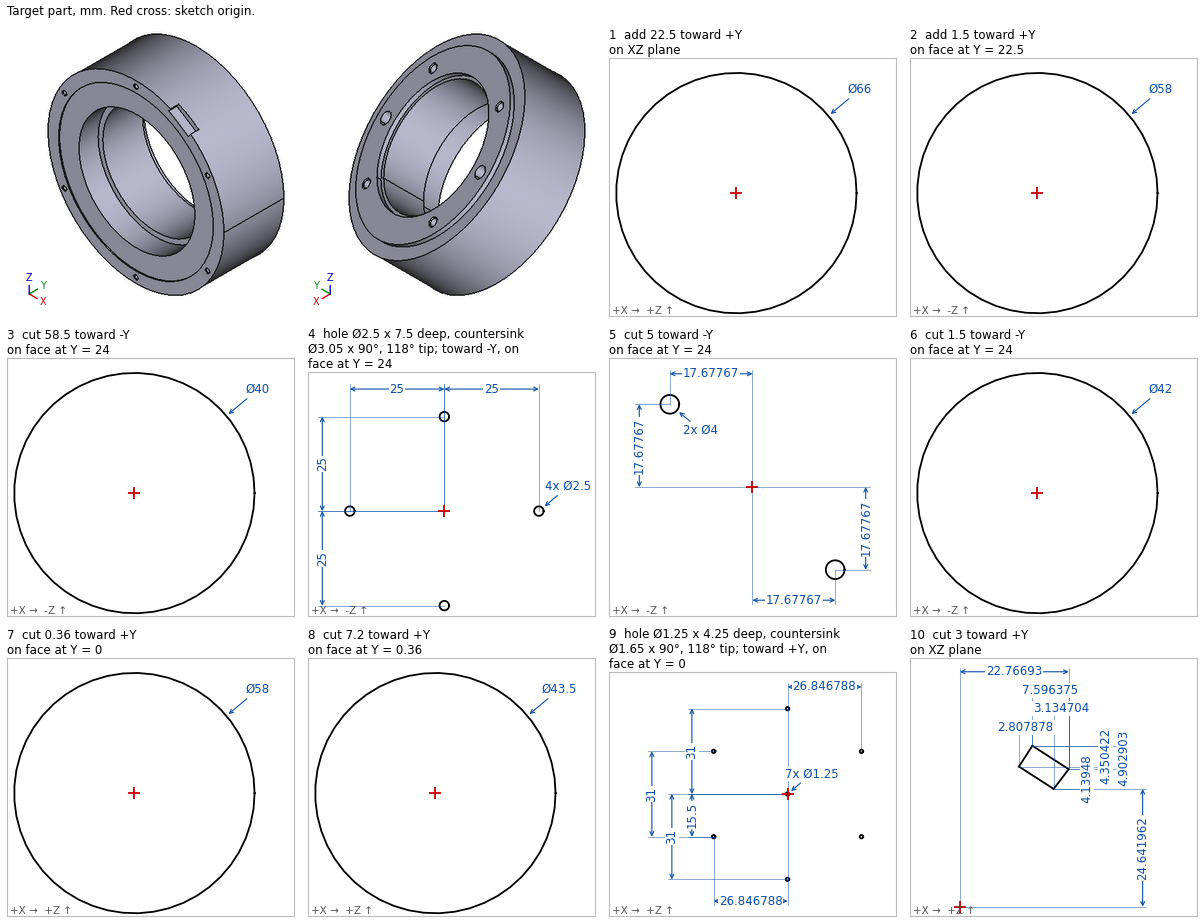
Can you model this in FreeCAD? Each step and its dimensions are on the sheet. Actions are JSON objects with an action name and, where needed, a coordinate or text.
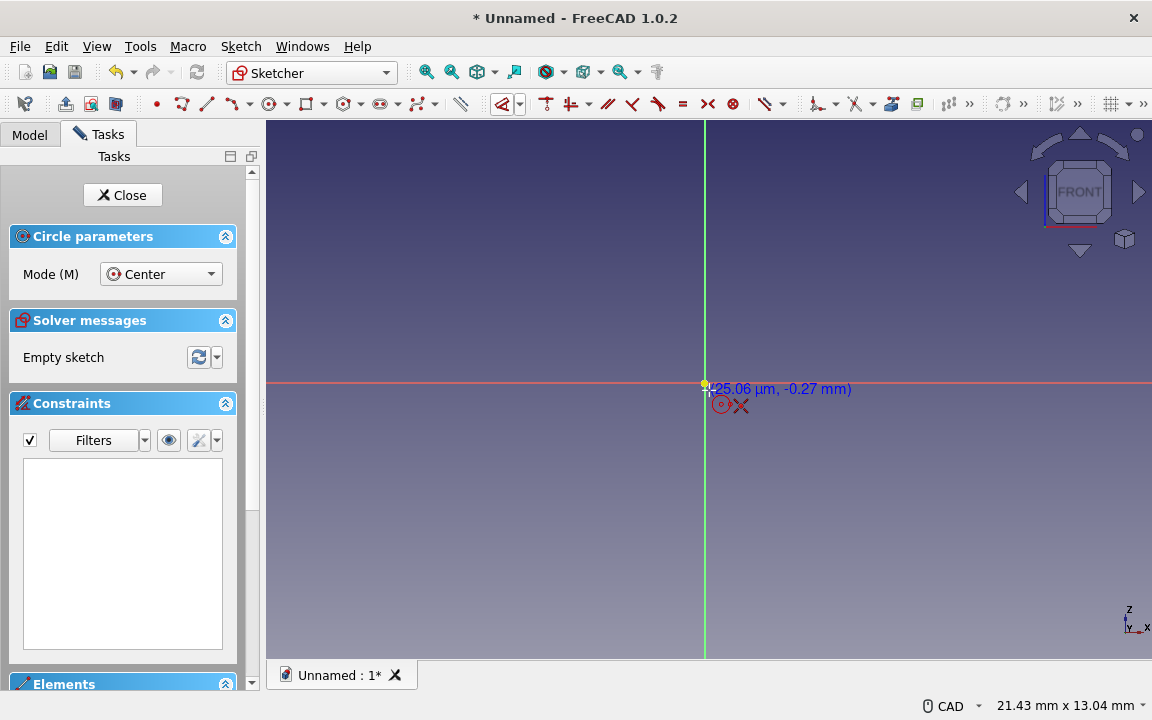
{"action": "scroll", "coordinate": [630, 391], "scroll_direction": "down", "scroll_amount": 10}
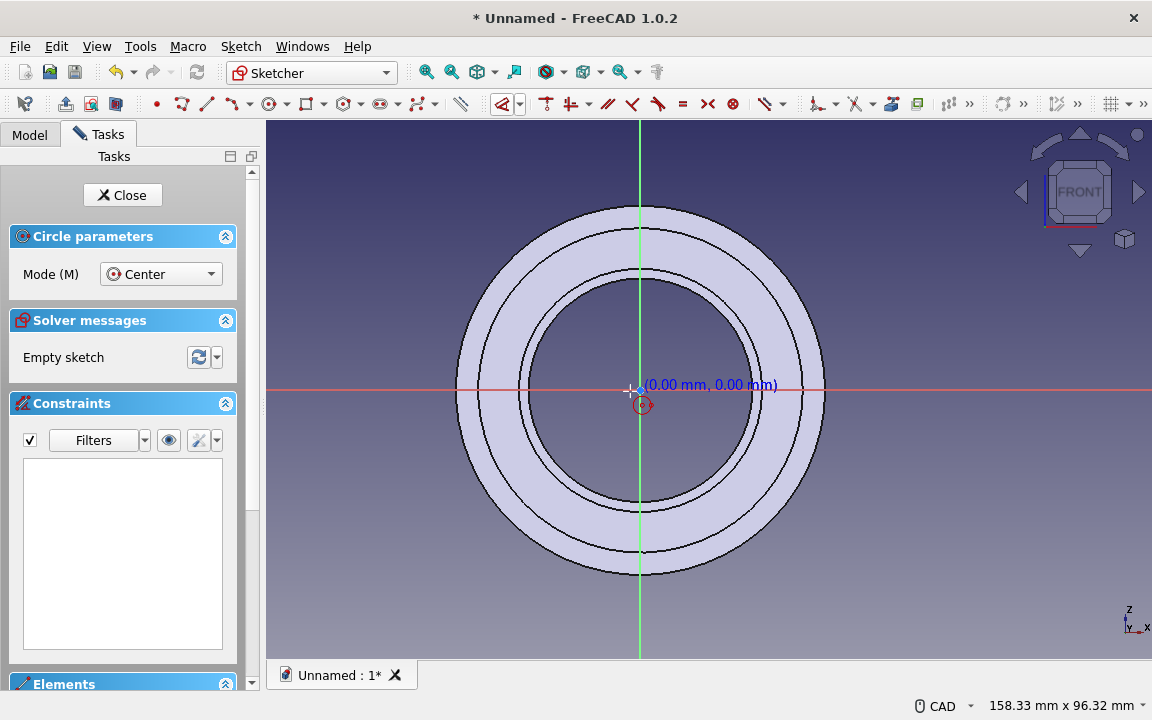
{"action": "left_click", "coordinate": [640, 390]}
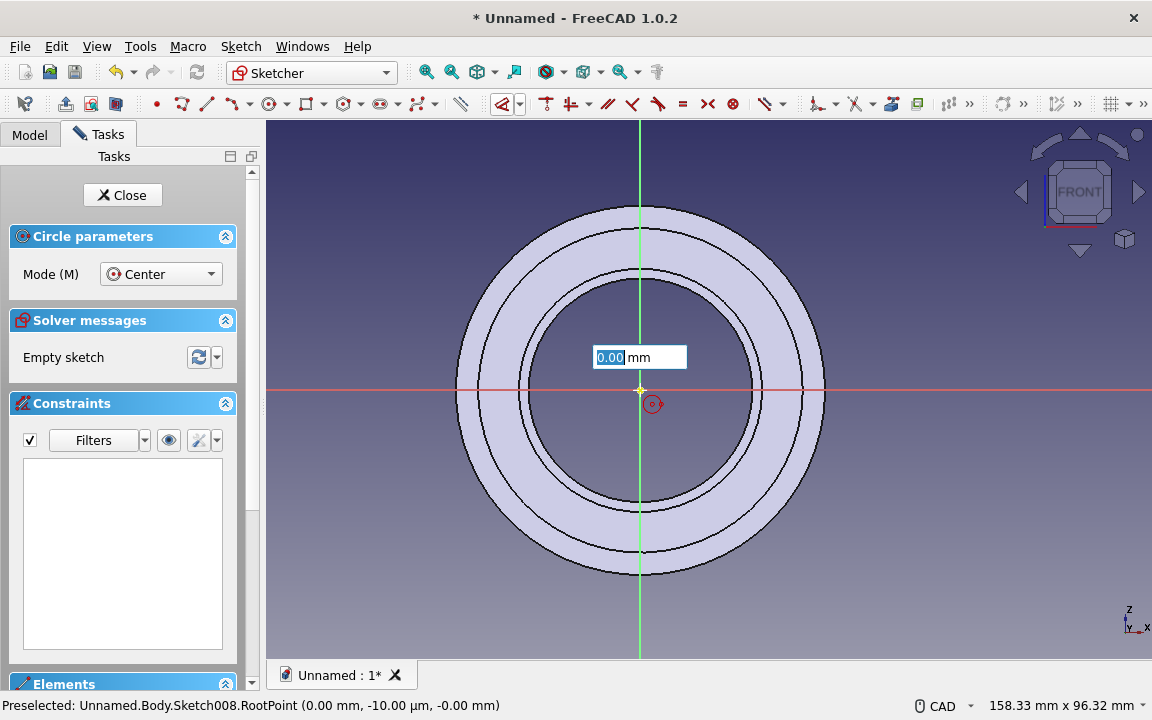
{"action": "scroll", "coordinate": [643, 388], "scroll_direction": "up", "scroll_amount": 10}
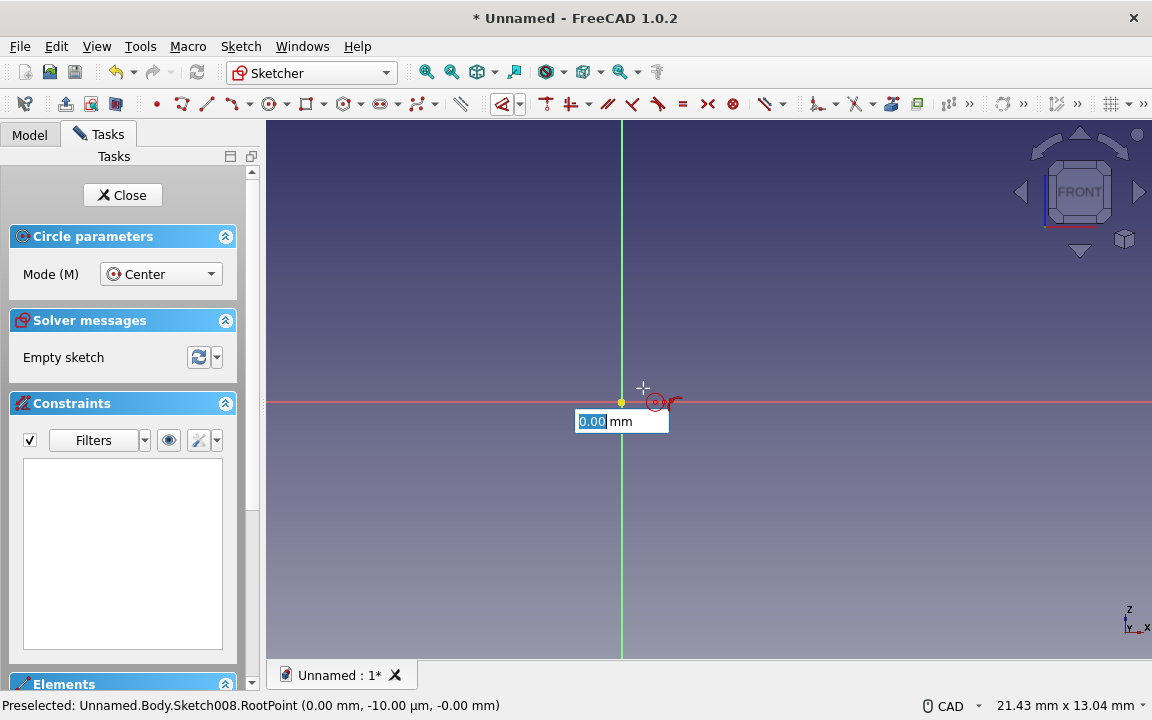
{"action": "left_click", "coordinate": [640, 384]}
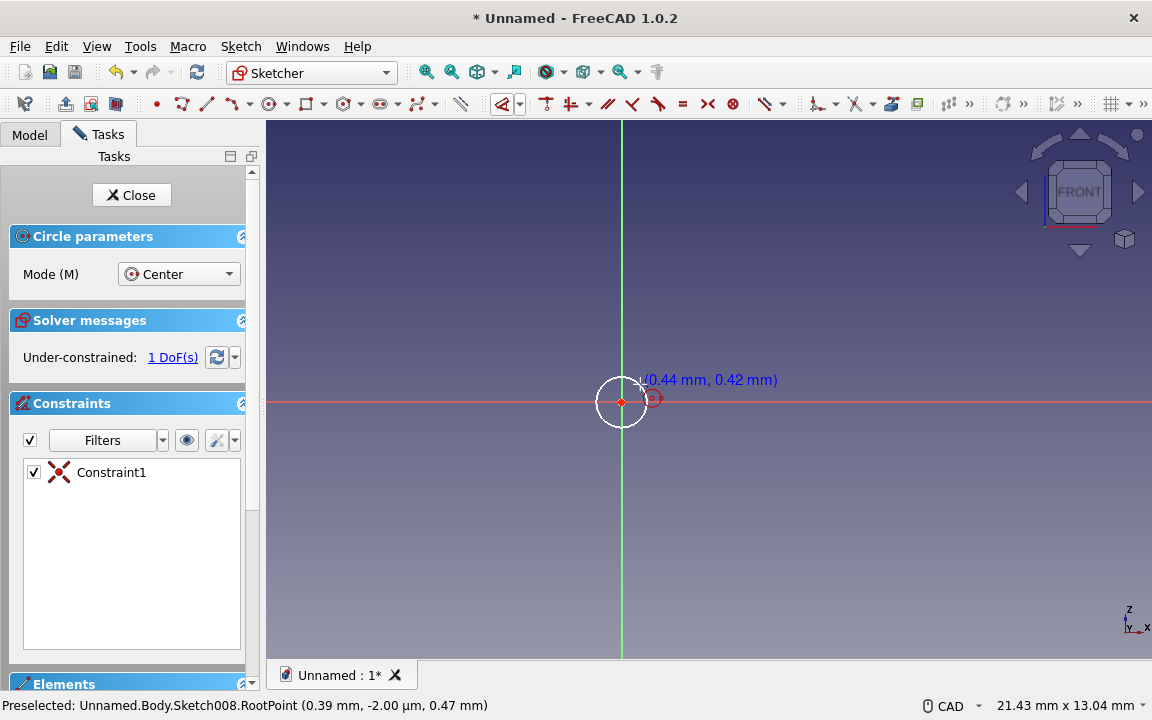
{"action": "scroll", "coordinate": [643, 387], "scroll_direction": "down", "scroll_amount": 10}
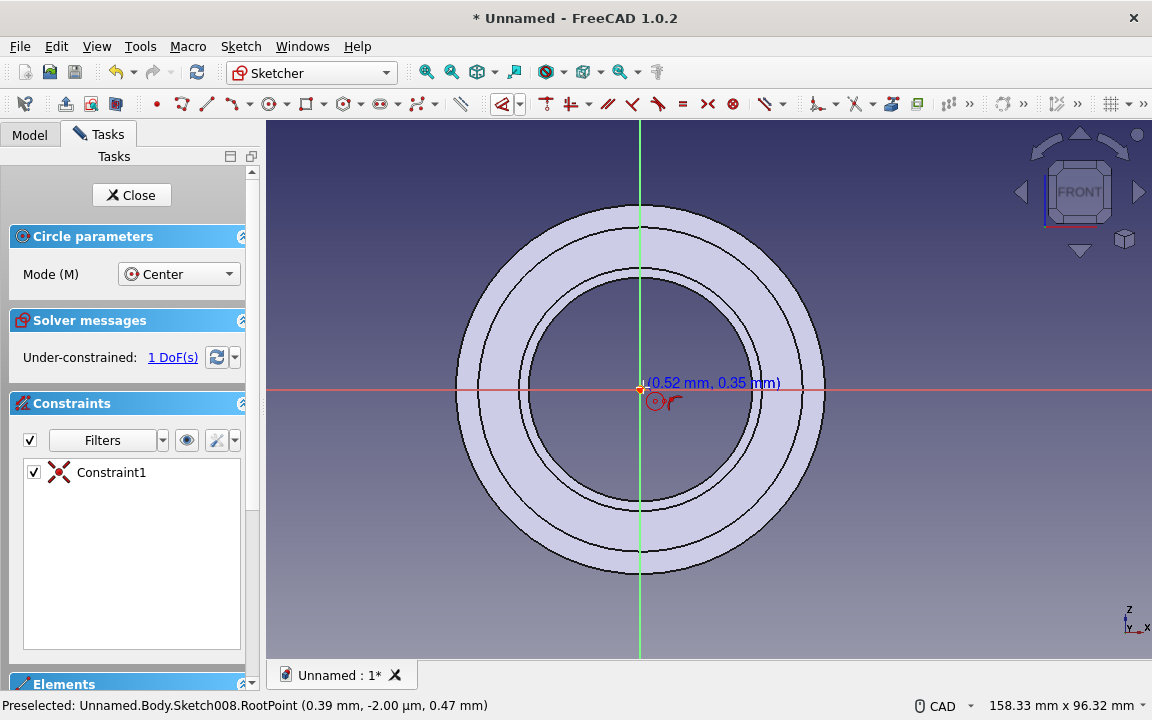
{"action": "scroll", "coordinate": [640, 563], "scroll_direction": "up", "scroll_amount": 10}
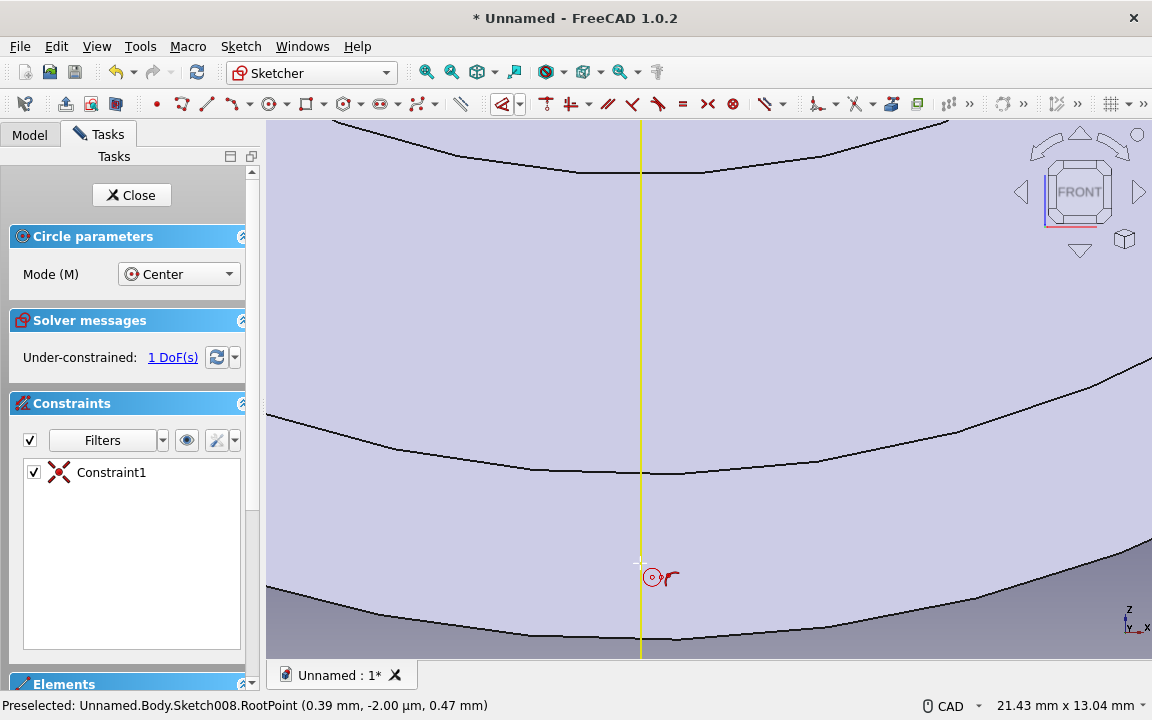
{"action": "scroll", "coordinate": [640, 564], "scroll_direction": "down", "scroll_amount": 10}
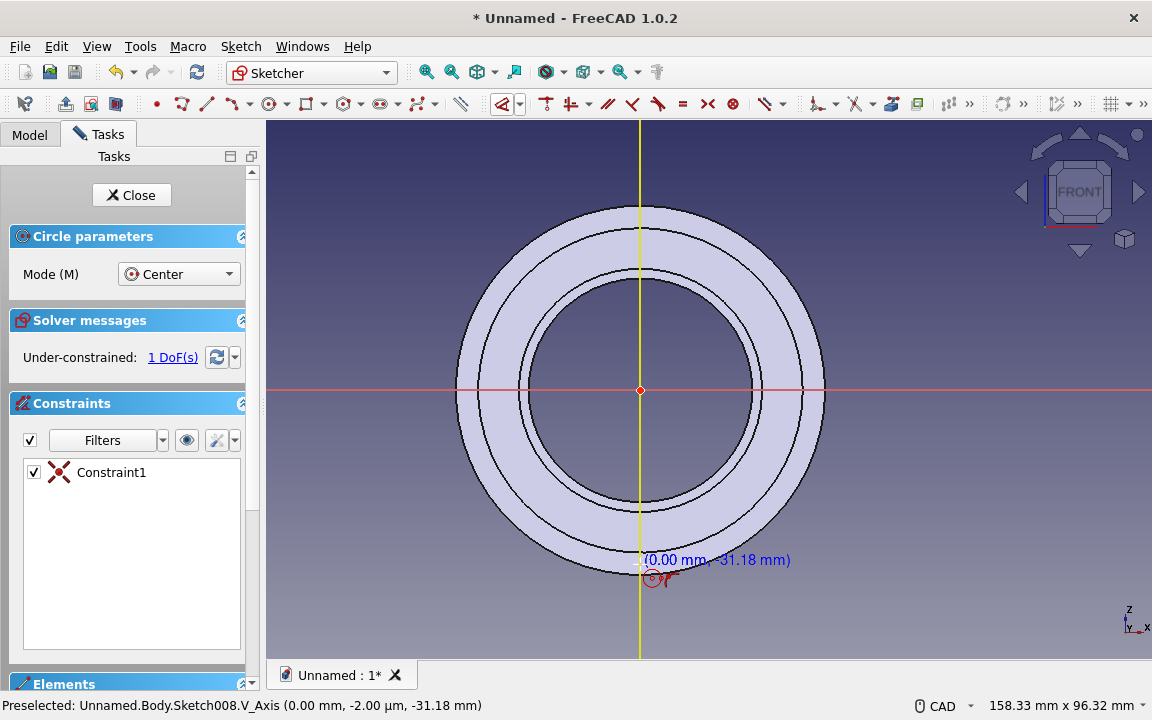
{"action": "left_click", "coordinate": [640, 564]}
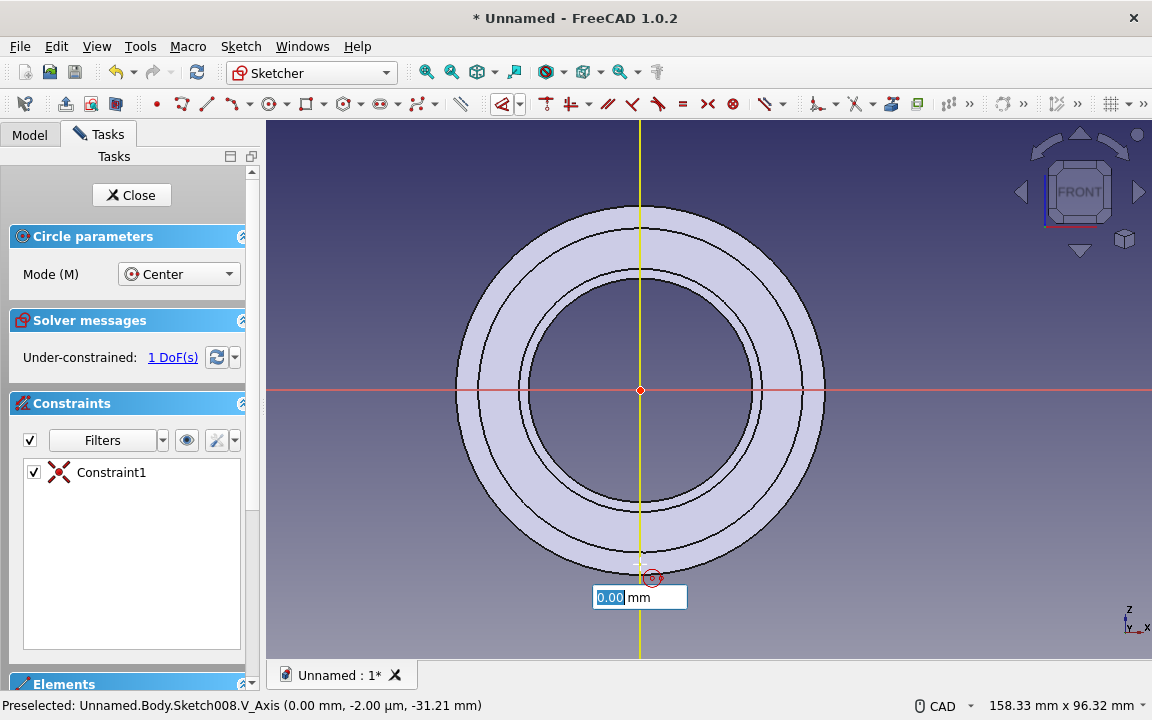
{"action": "scroll", "coordinate": [644, 563], "scroll_direction": "up", "scroll_amount": 8}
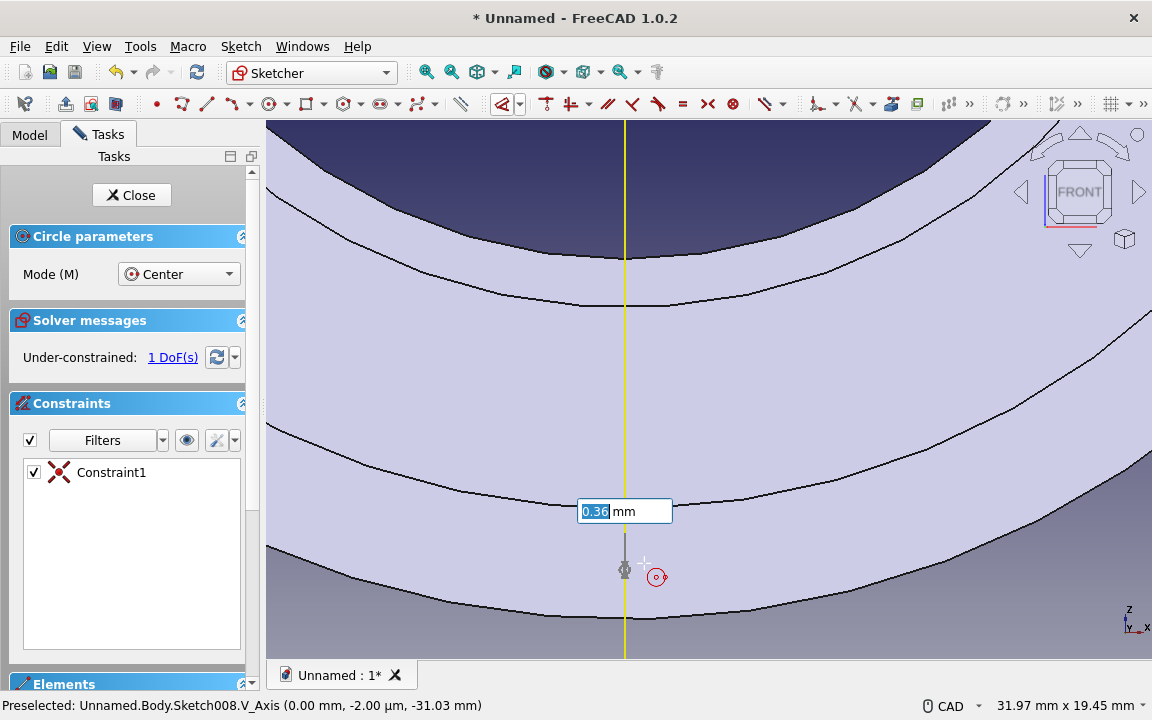
{"action": "left_click", "coordinate": [641, 558]}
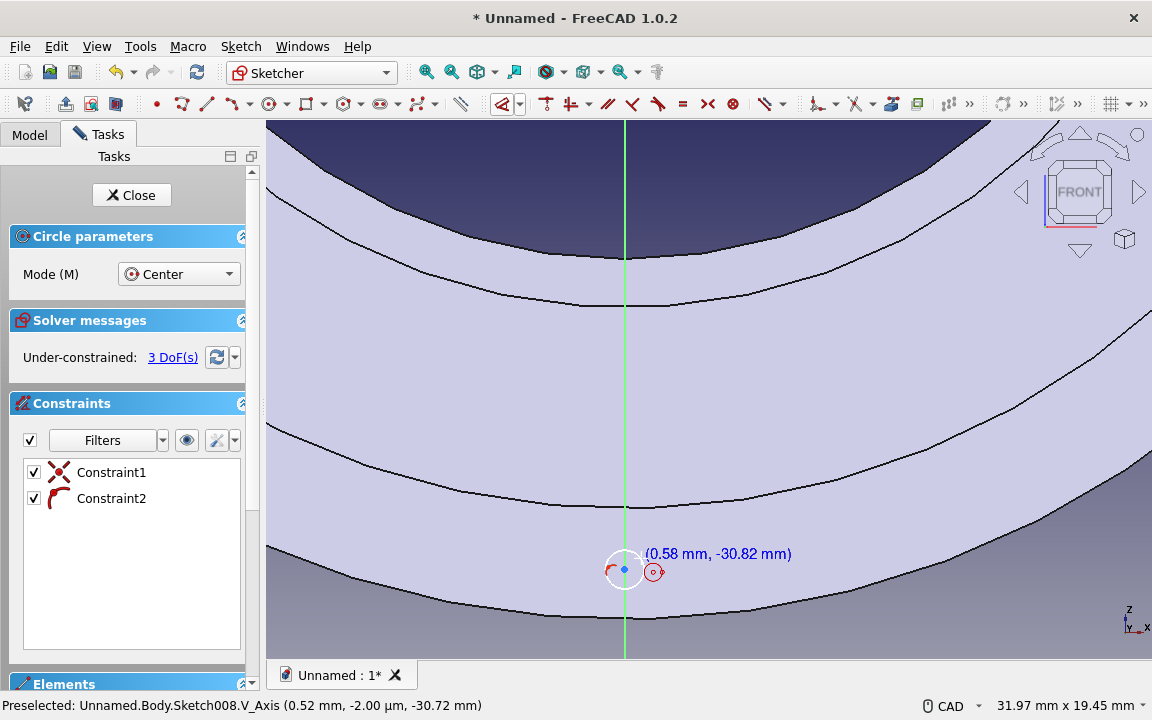
{"action": "scroll", "coordinate": [644, 563], "scroll_direction": "down", "scroll_amount": 8}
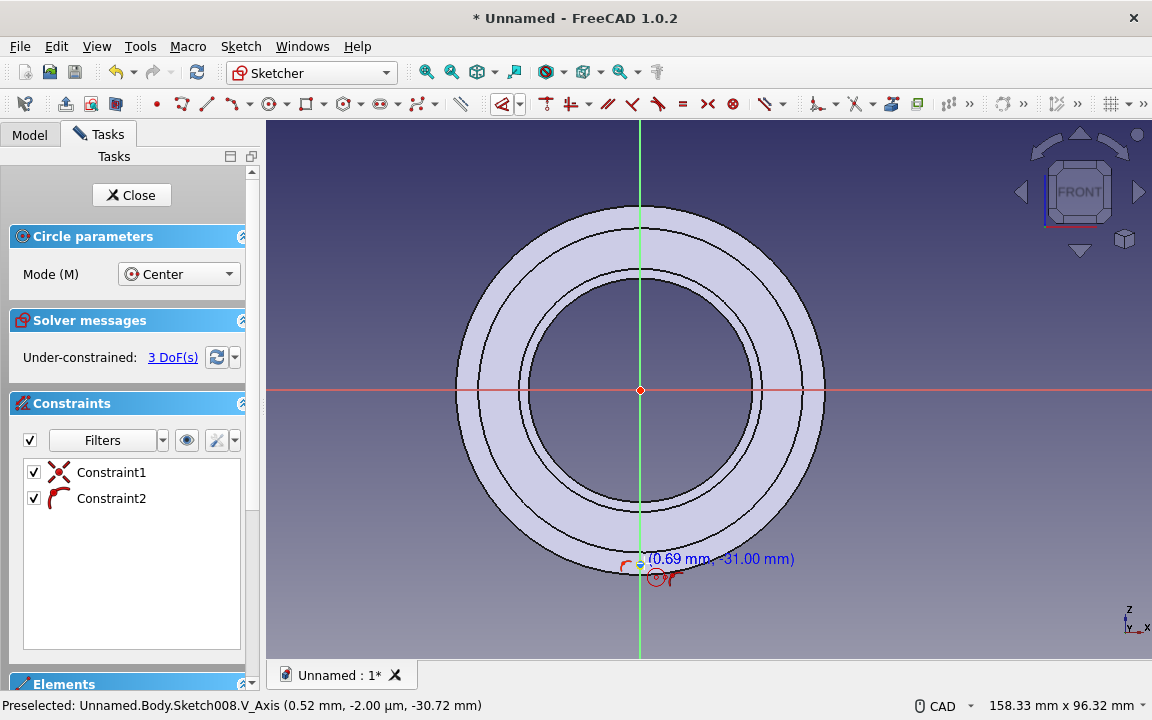
{"action": "scroll", "coordinate": [490, 477], "scroll_direction": "up", "scroll_amount": 10}